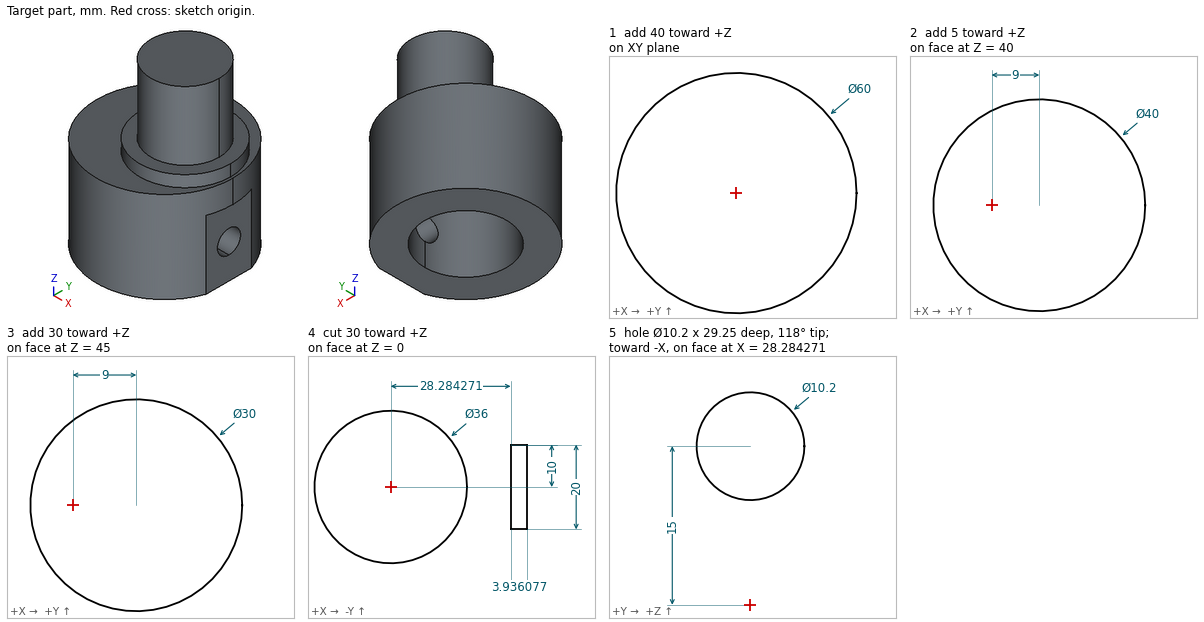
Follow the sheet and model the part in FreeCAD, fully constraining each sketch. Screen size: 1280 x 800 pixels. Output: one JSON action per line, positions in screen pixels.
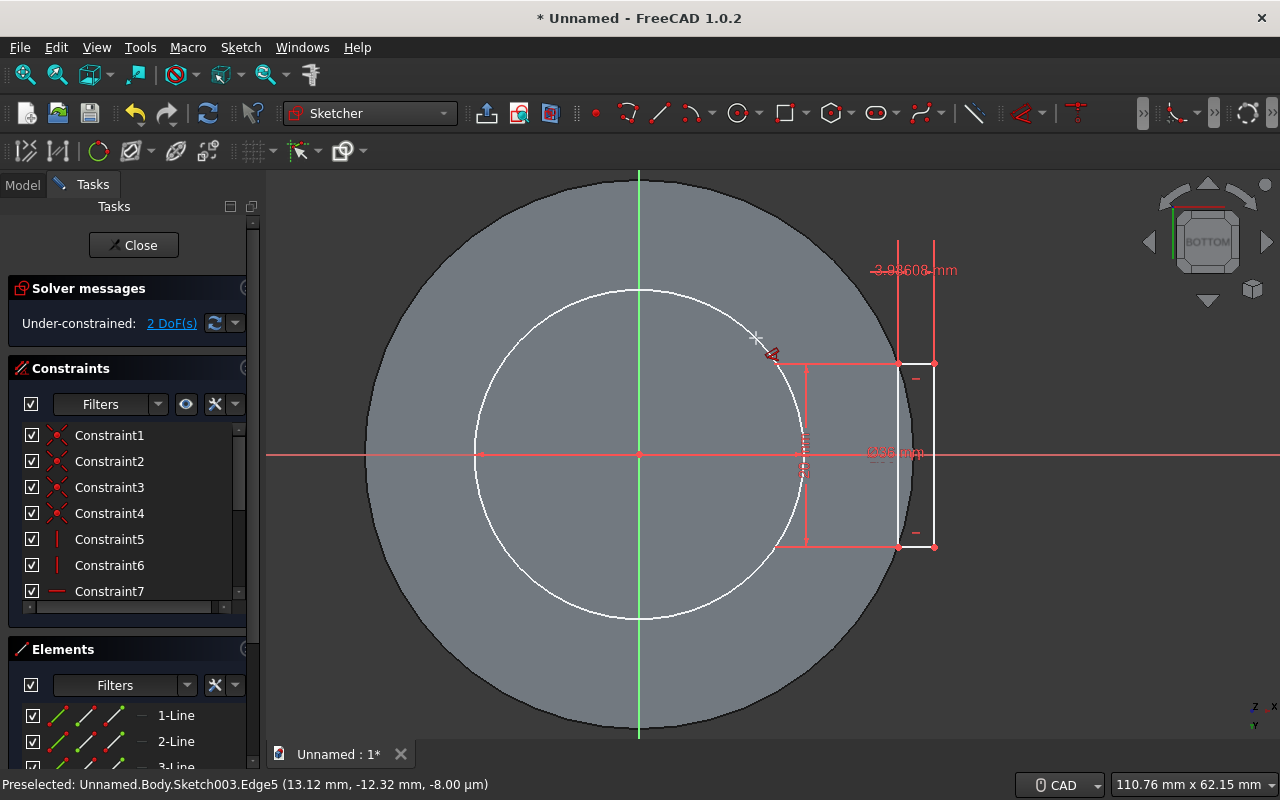
{"action": "left_click", "coordinate": [898, 364]}
{"action": "left_click", "coordinate": [605, 409]}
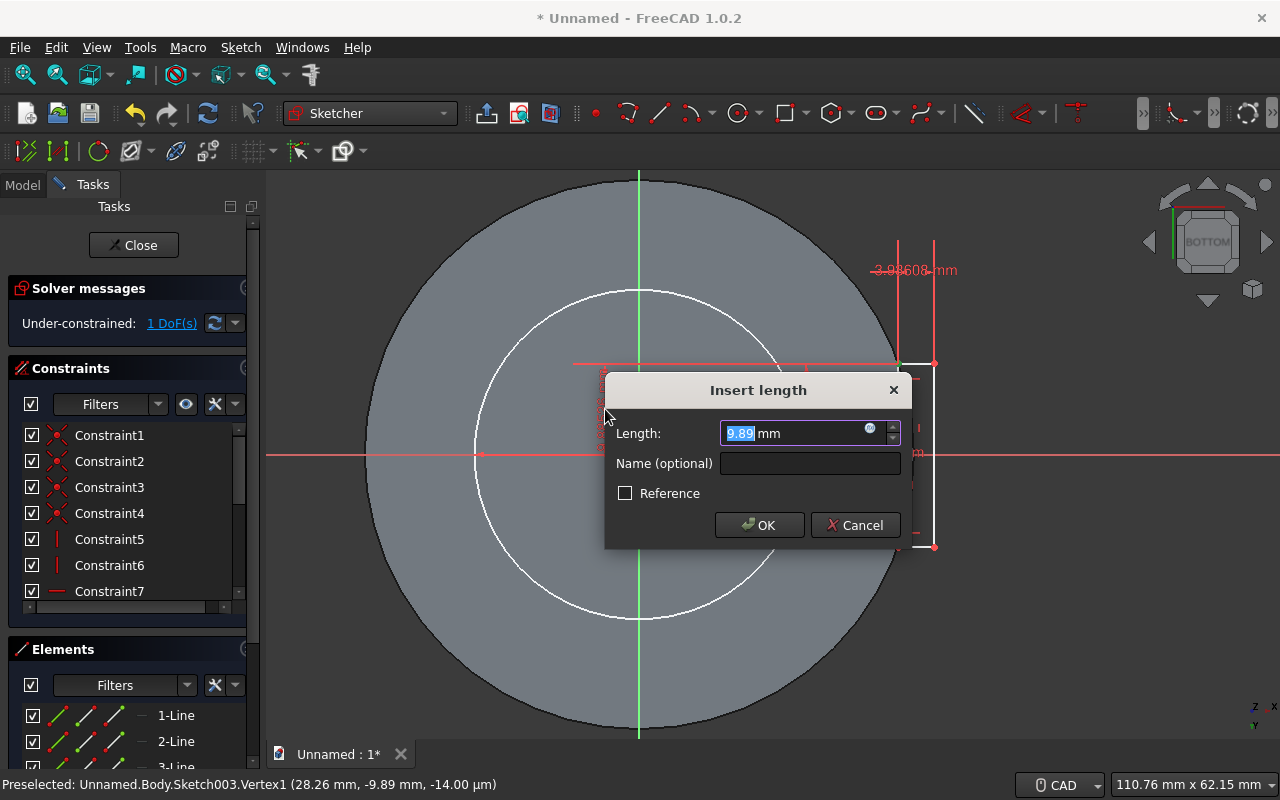
{"action": "type", "text": "10"}
{"action": "key", "text": "Return"}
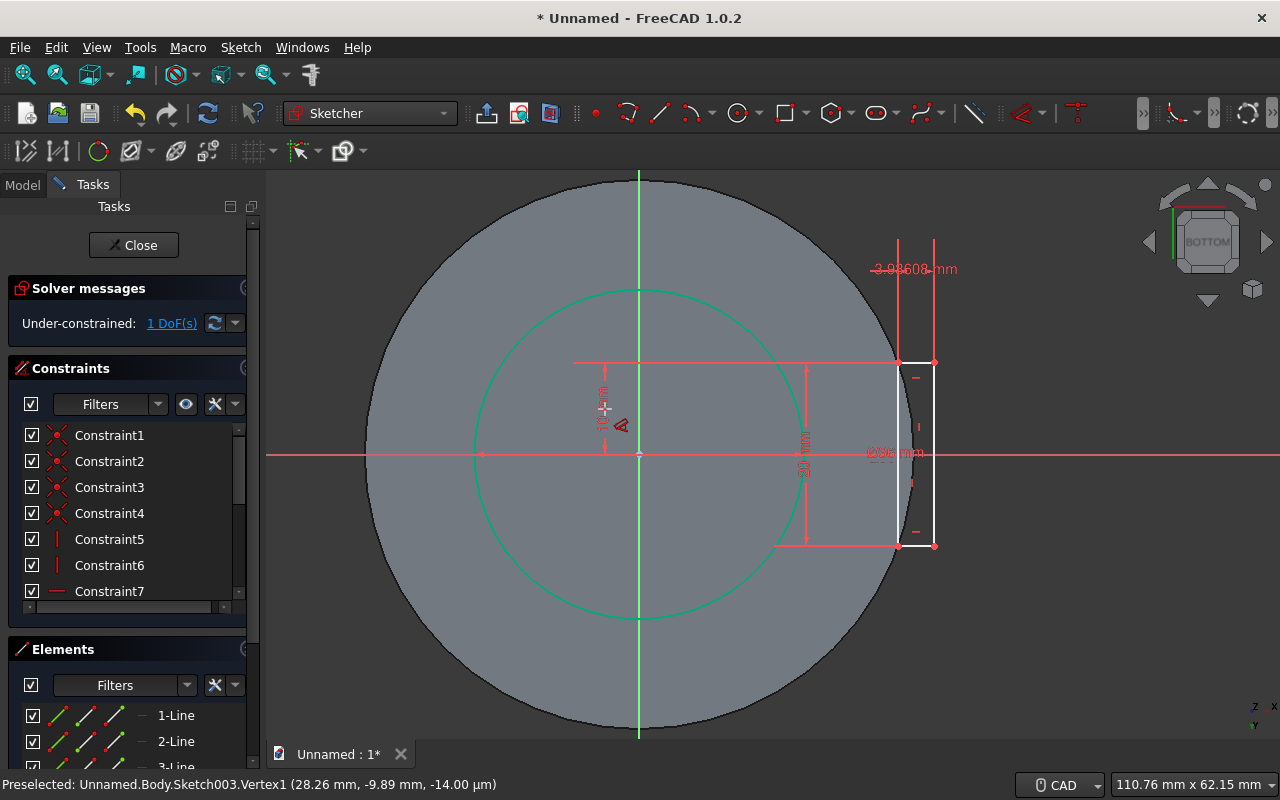
{"action": "left_click", "coordinate": [898, 363]}
{"action": "left_click", "coordinate": [769, 329]}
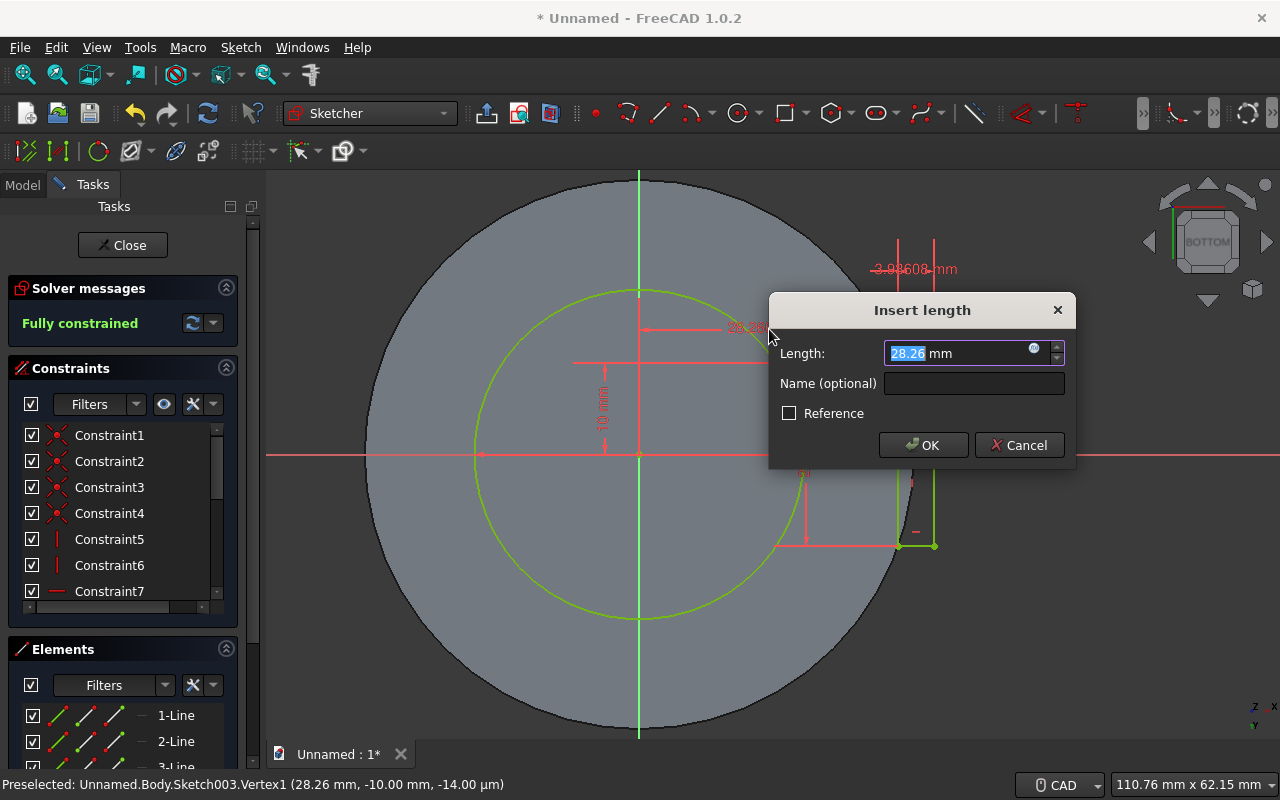
{"action": "type", "text": "28.284271"}
{"action": "key", "text": "Return"}
{"action": "key", "text": "Escape"}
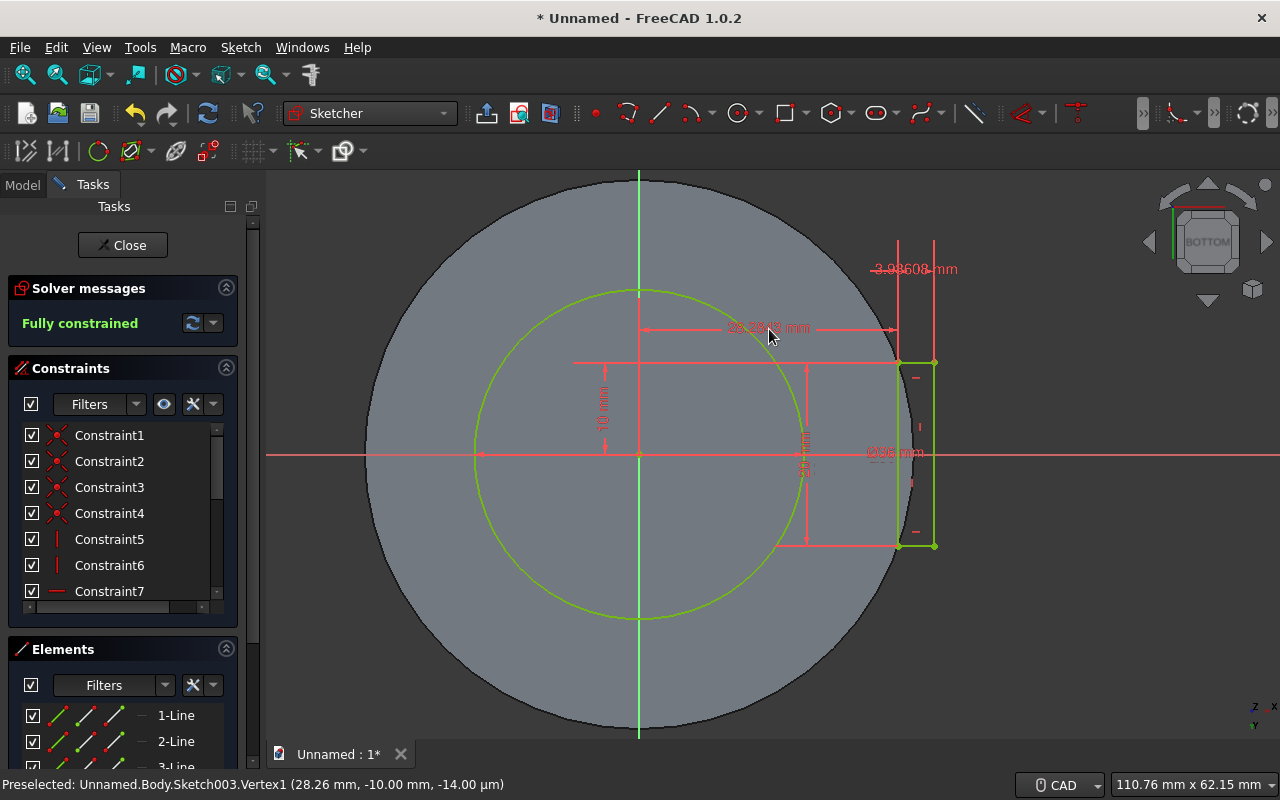
{"action": "left_click", "coordinate": [123, 245]}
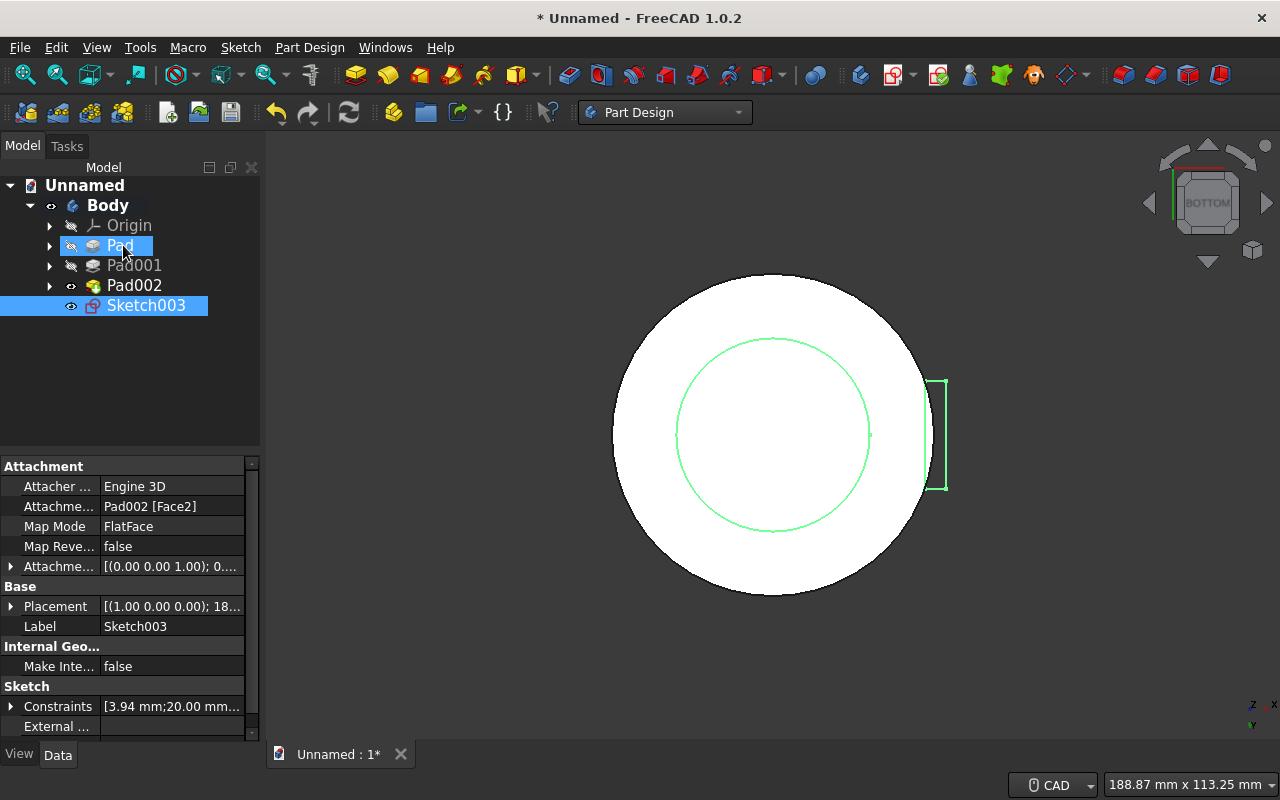
{"action": "left_click", "coordinate": [570, 76]}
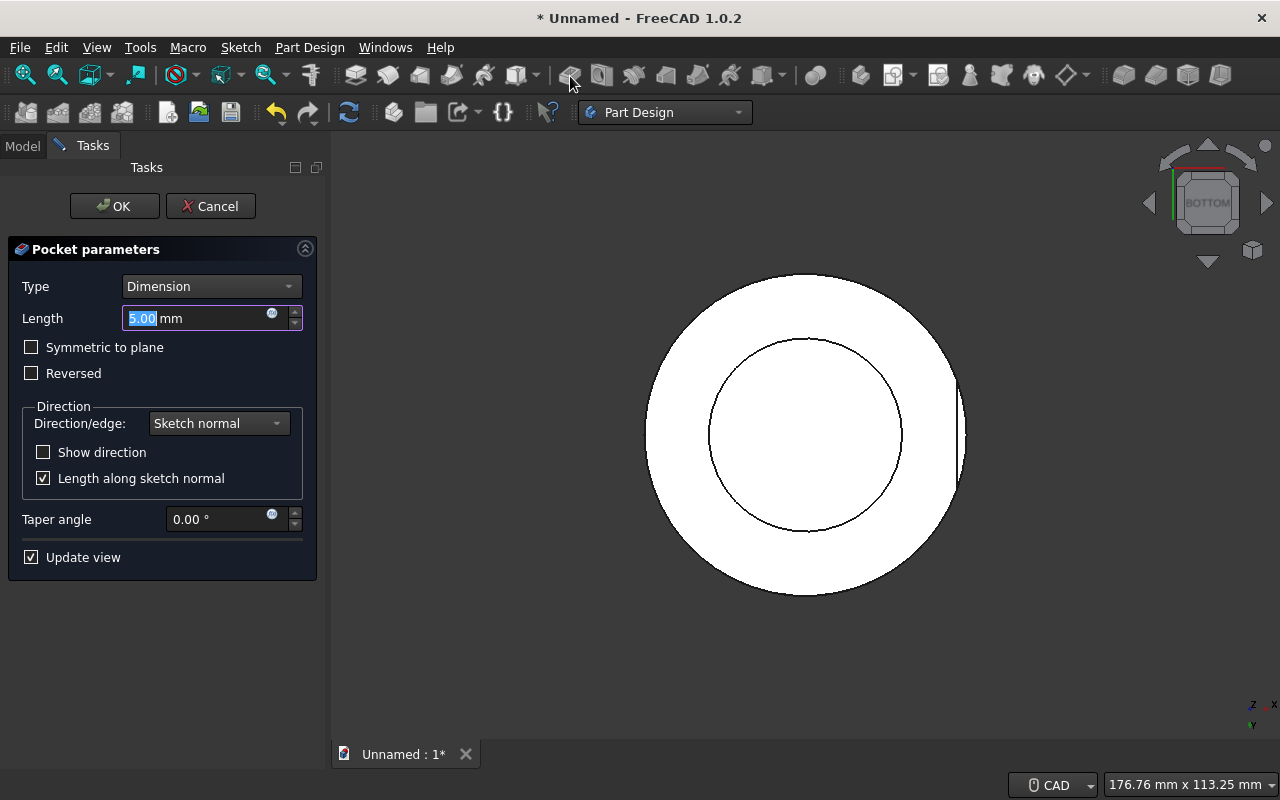
{"action": "type", "text": "30"}
{"action": "key", "text": "Tab"}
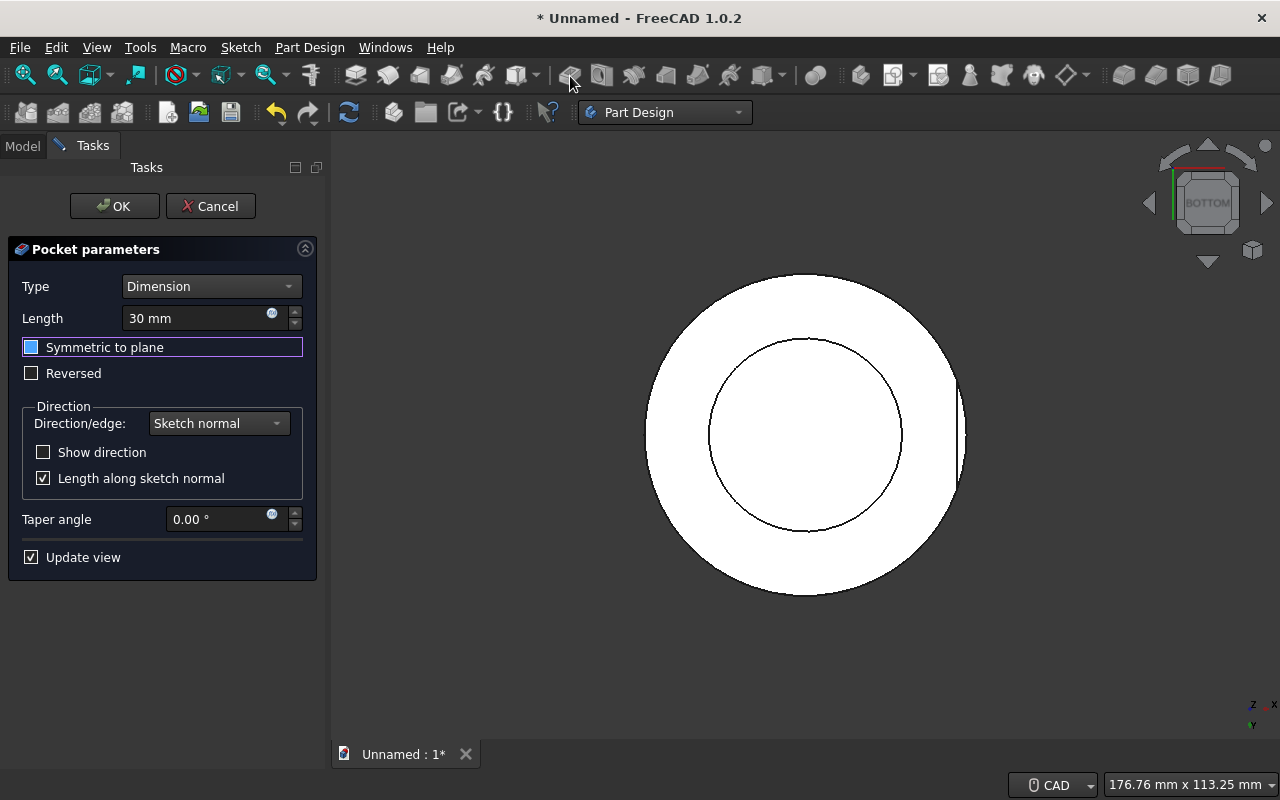
{"action": "left_click", "coordinate": [115, 206]}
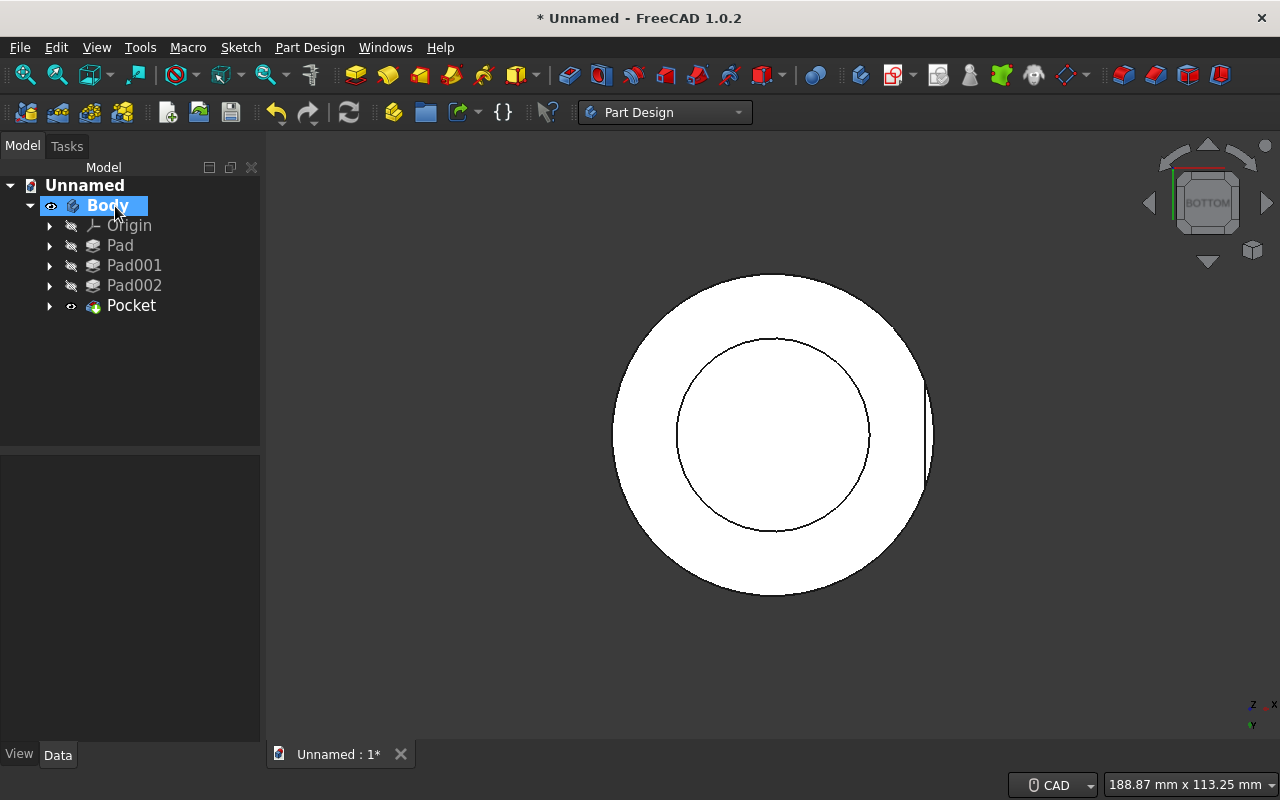
{"action": "key", "text": "0"}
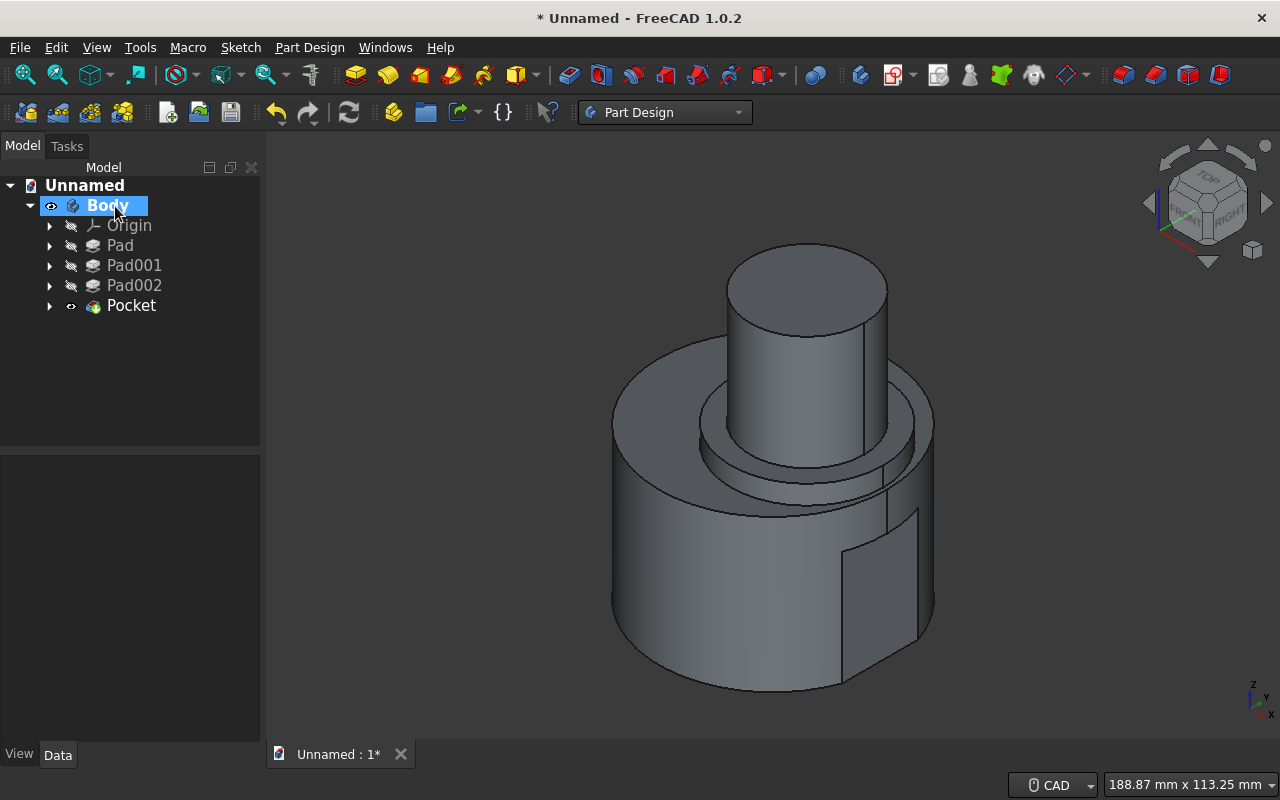
{"action": "left_click", "coordinate": [880, 576]}